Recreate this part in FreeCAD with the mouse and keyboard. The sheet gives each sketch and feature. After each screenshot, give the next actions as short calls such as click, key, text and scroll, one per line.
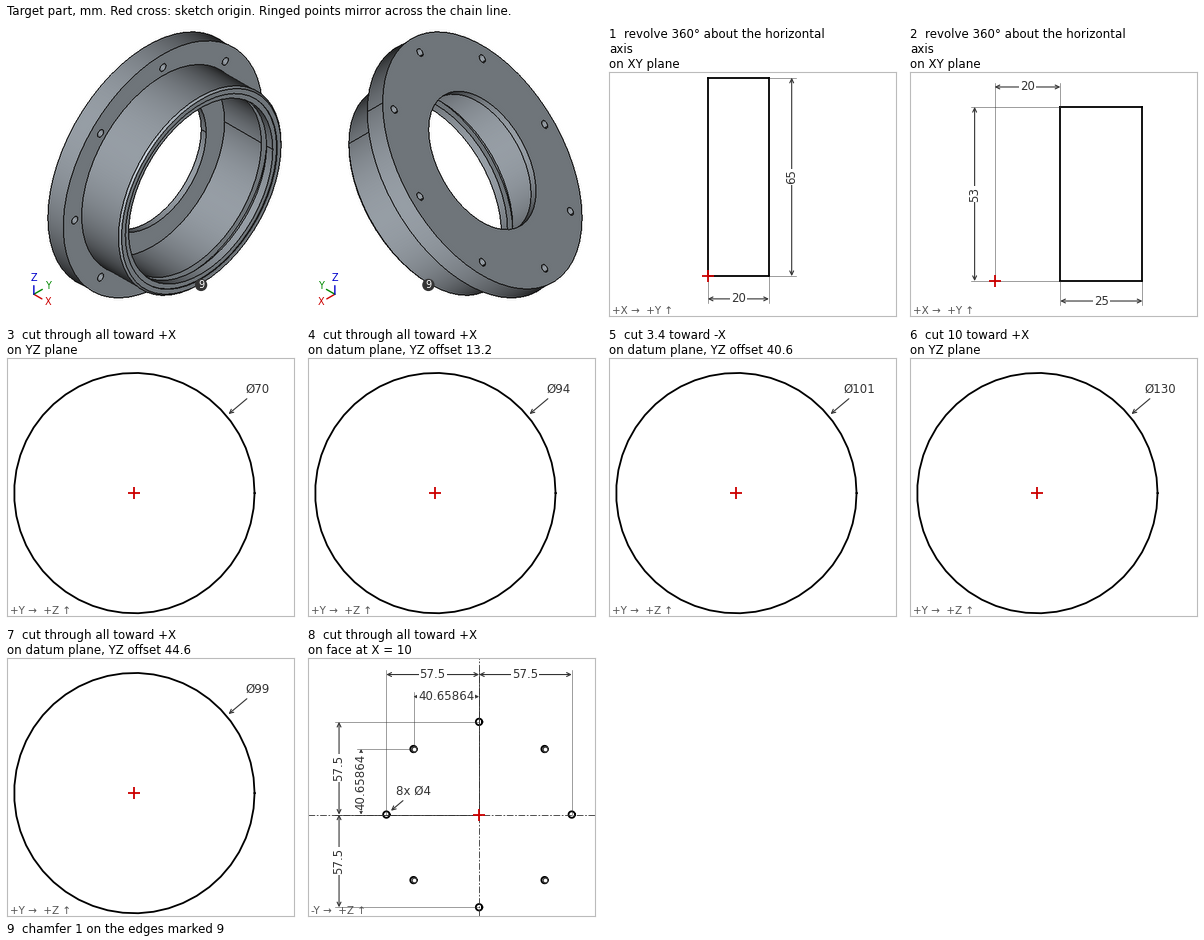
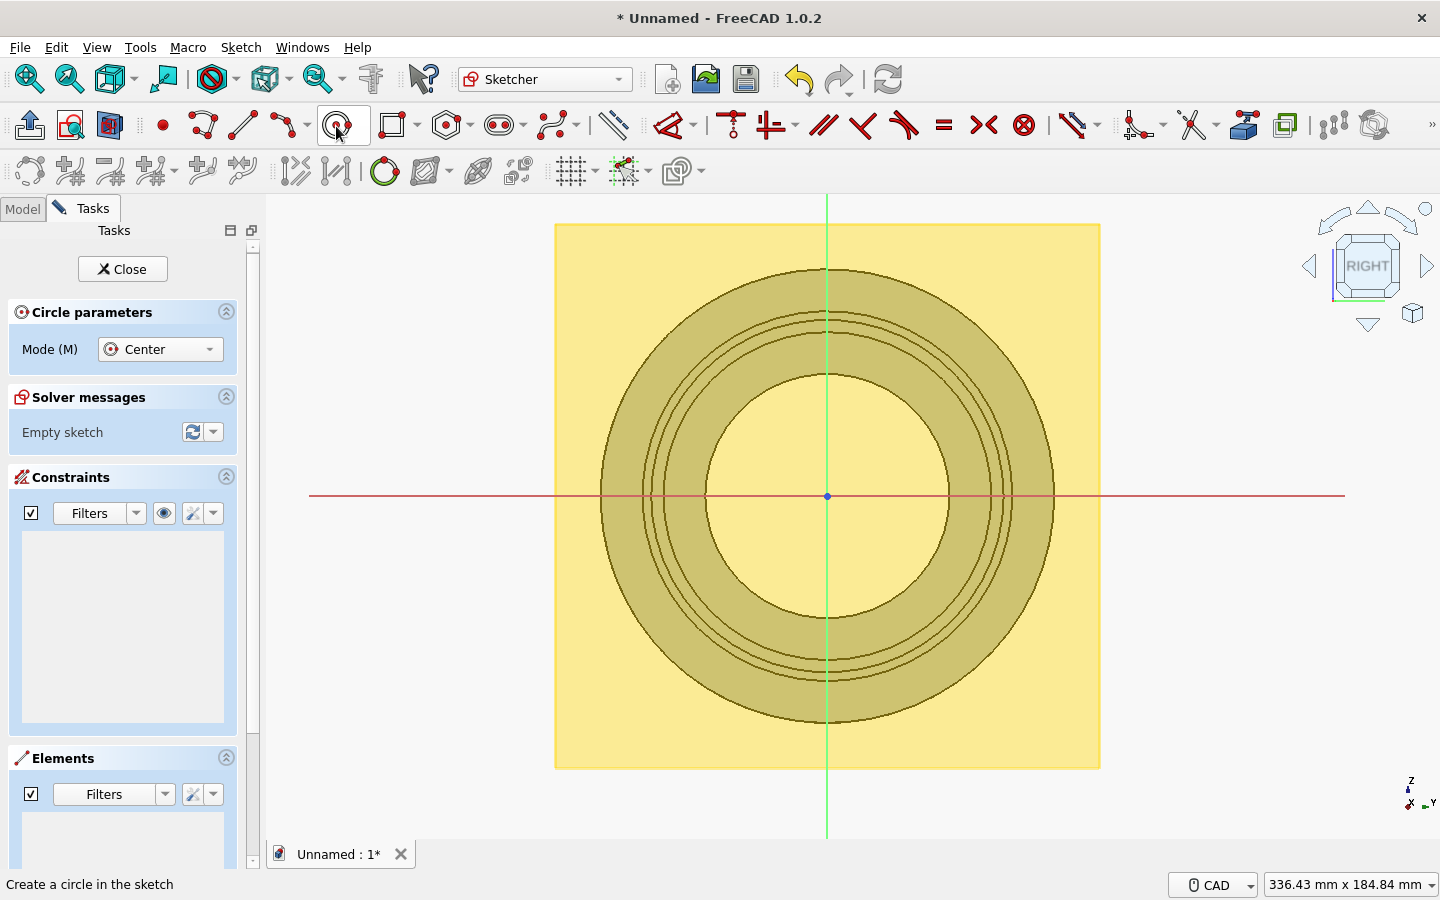
click(827, 496)
click(950, 374)
key(Escape)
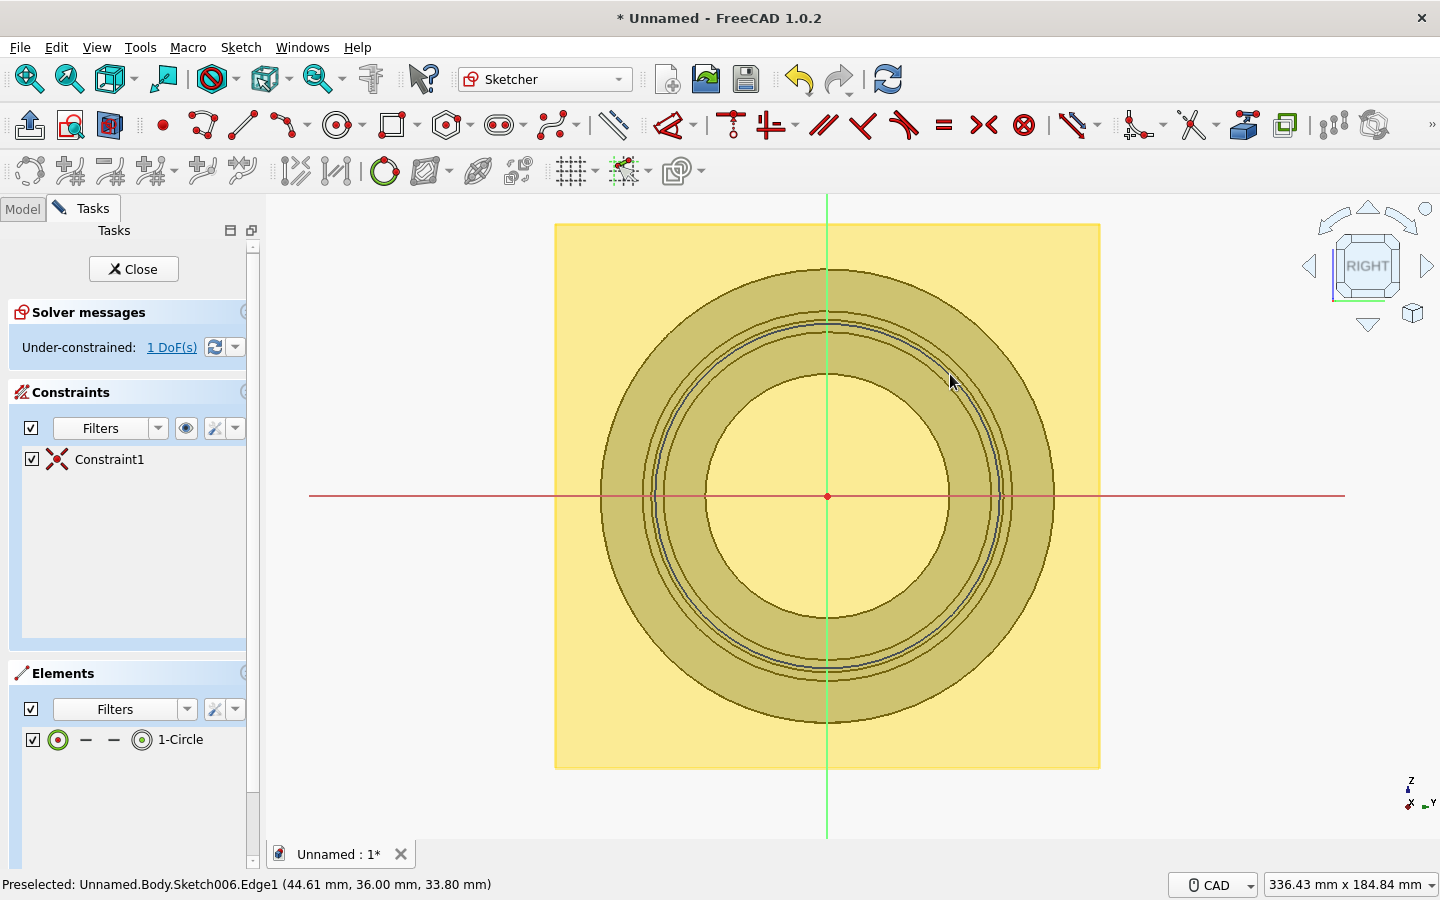
click(668, 126)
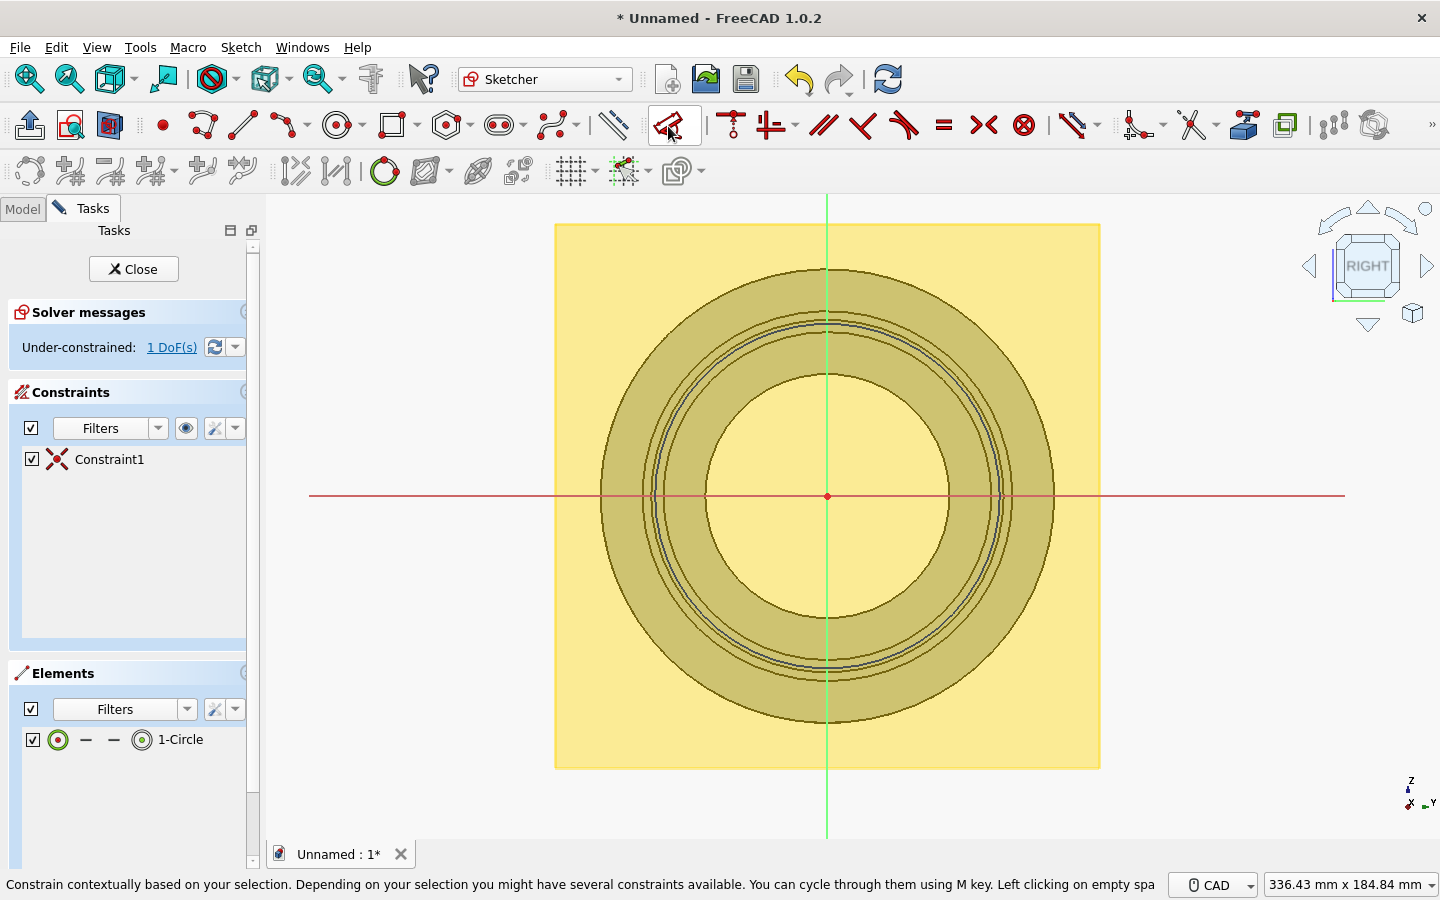
click(949, 374)
click(972, 351)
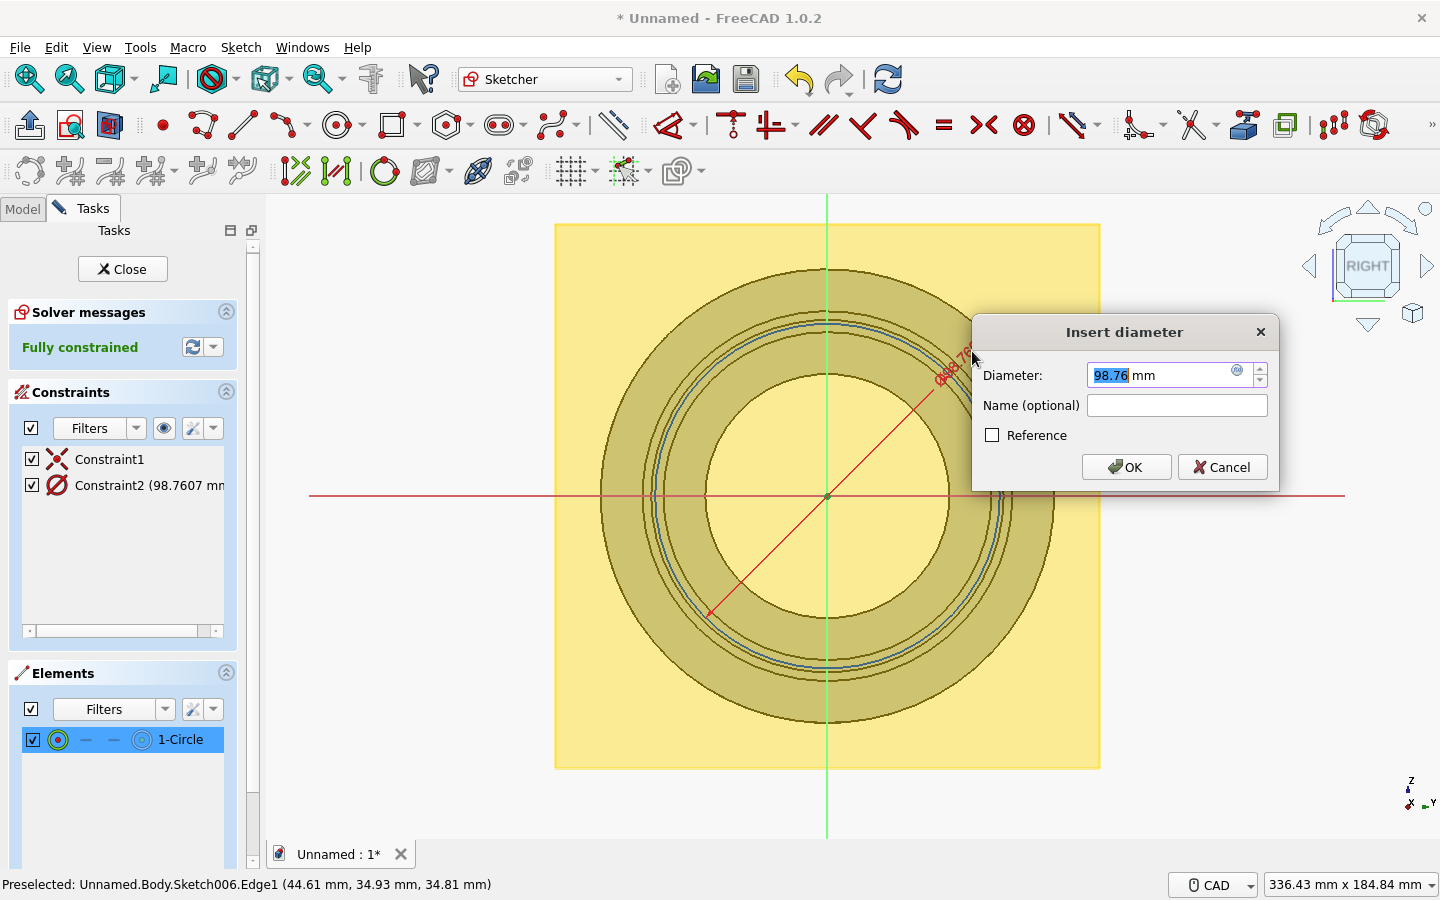
text(99)
key(Return)
key(Escape)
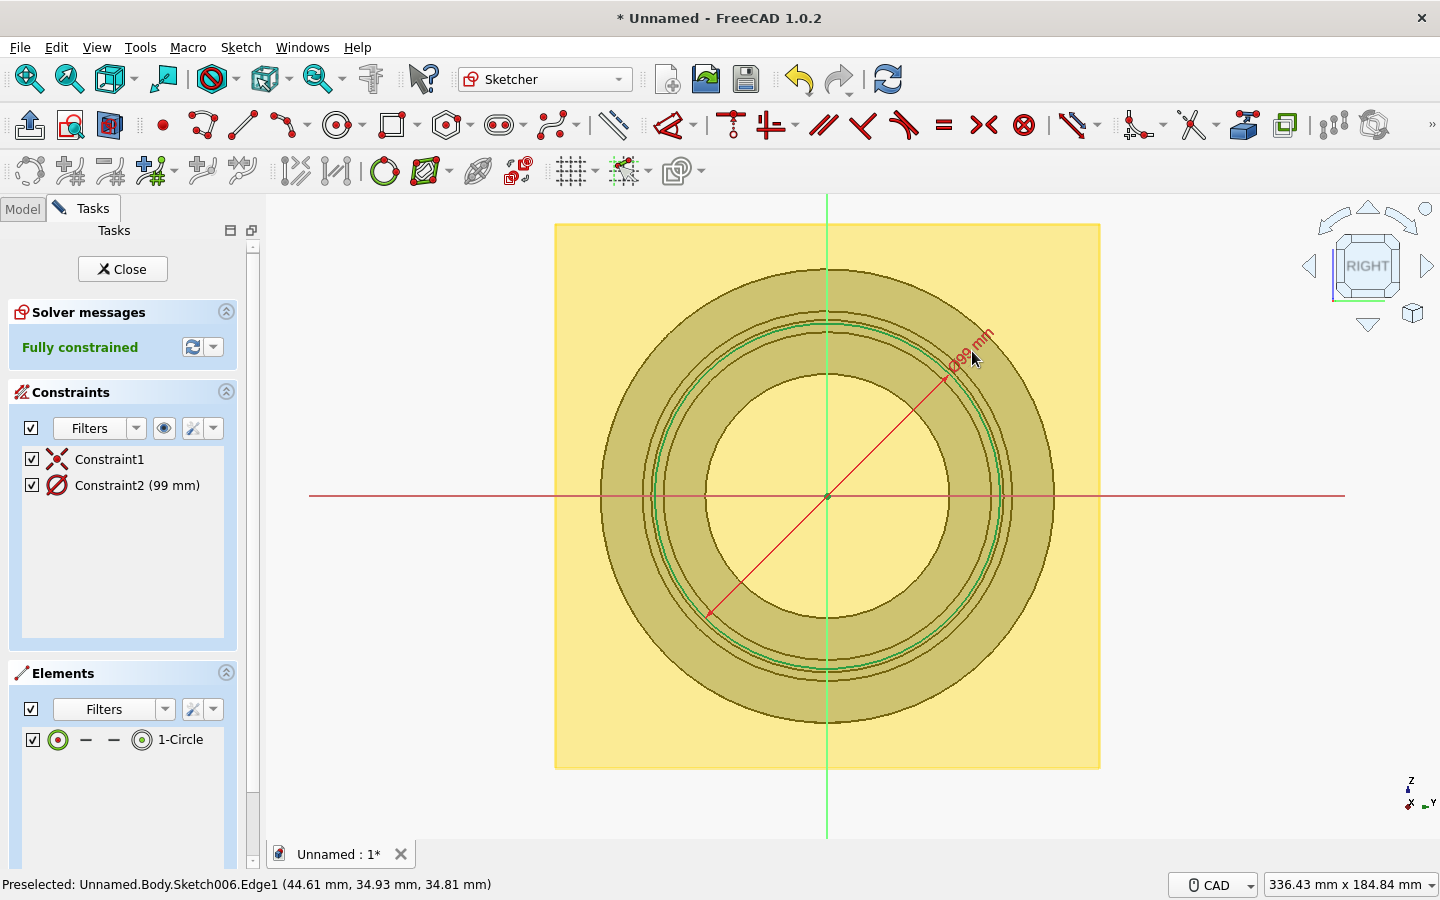
click(123, 269)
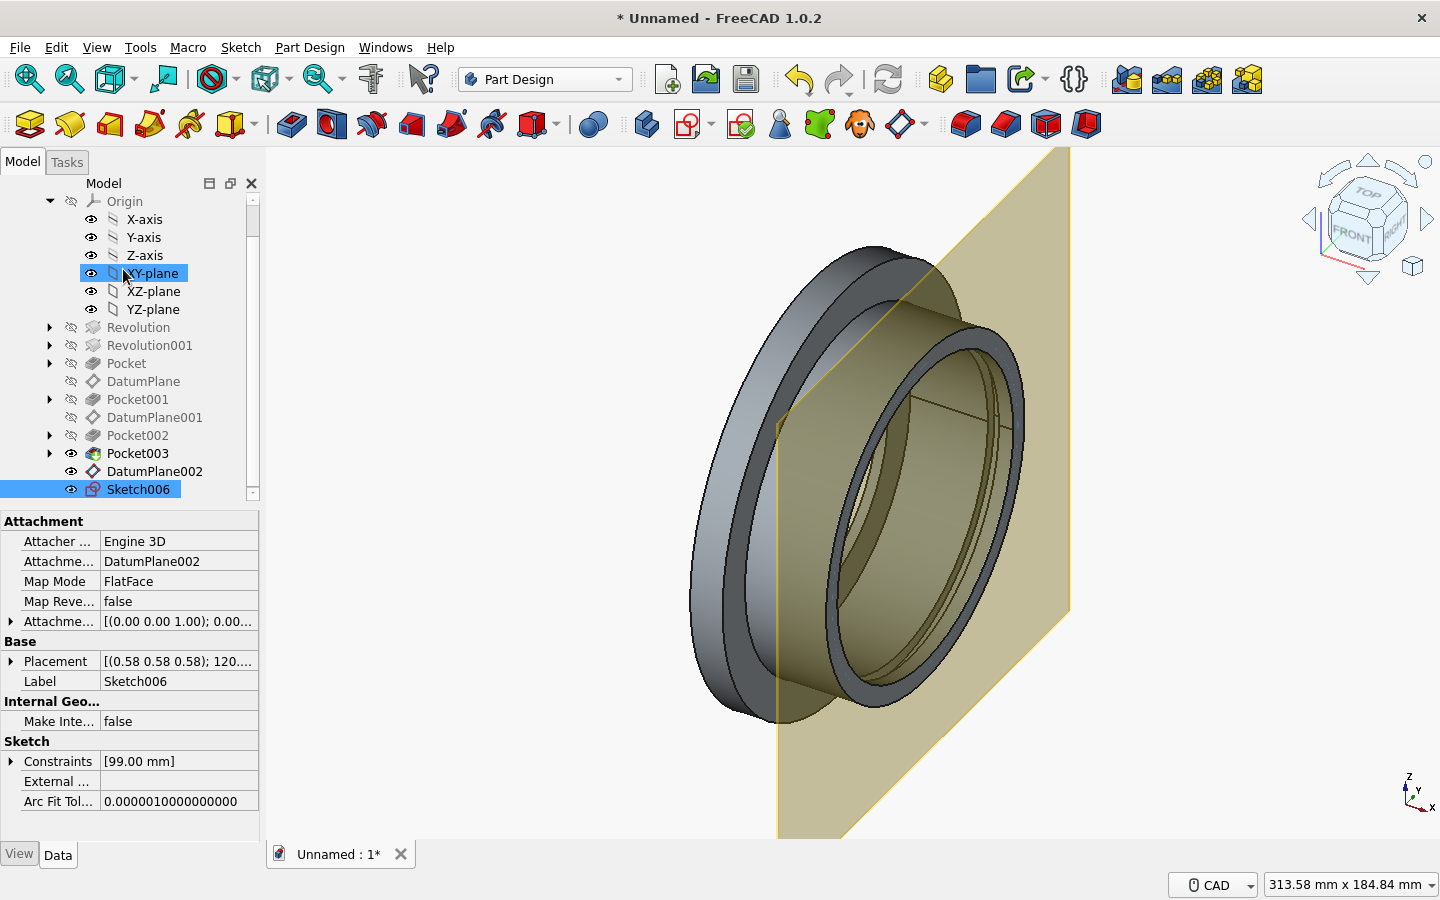
click(292, 124)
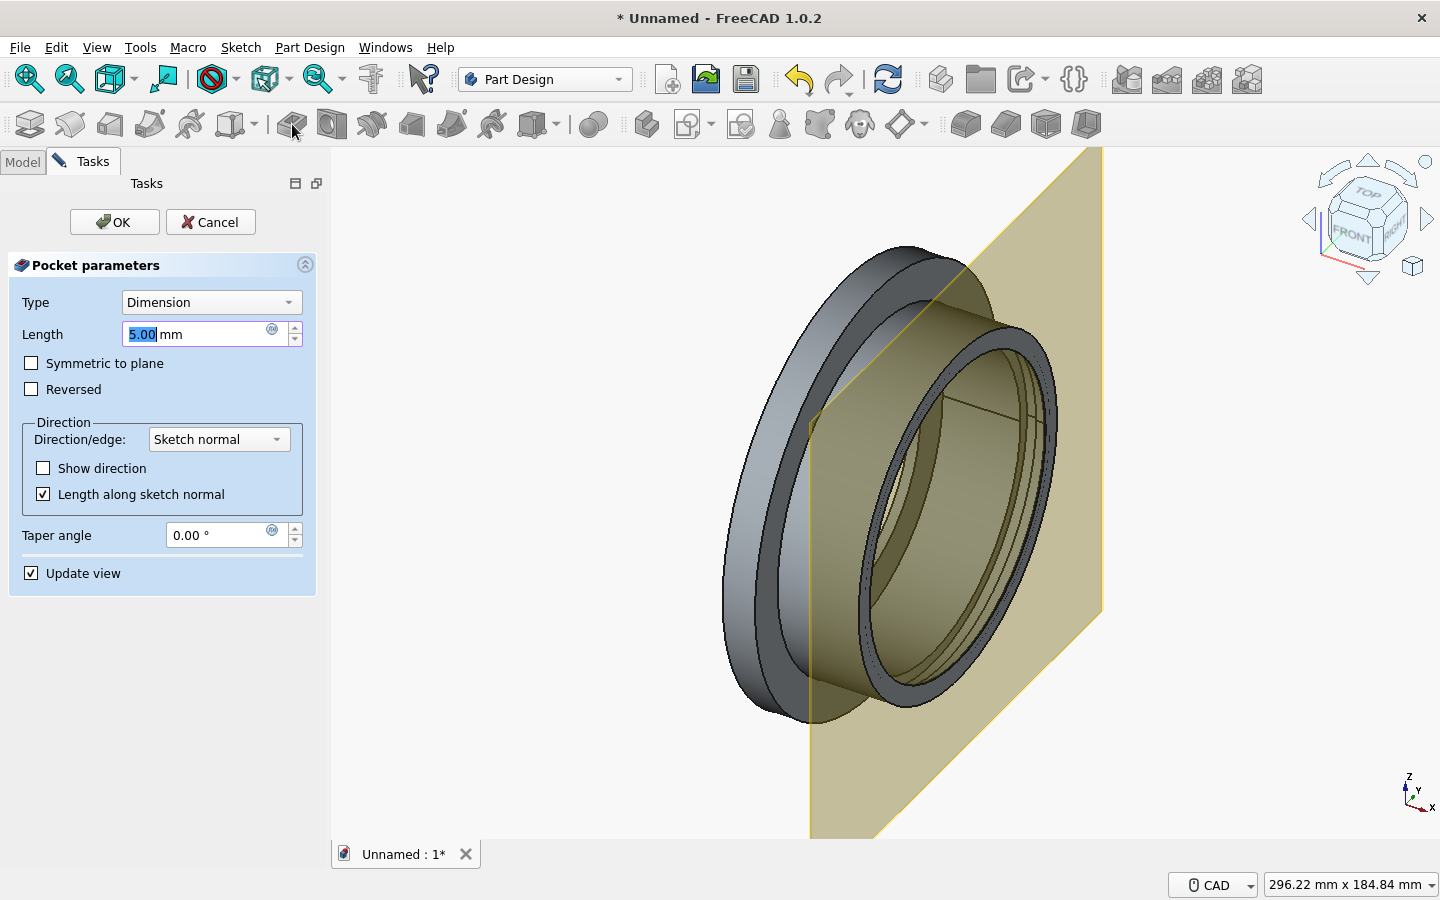
click(212, 302)